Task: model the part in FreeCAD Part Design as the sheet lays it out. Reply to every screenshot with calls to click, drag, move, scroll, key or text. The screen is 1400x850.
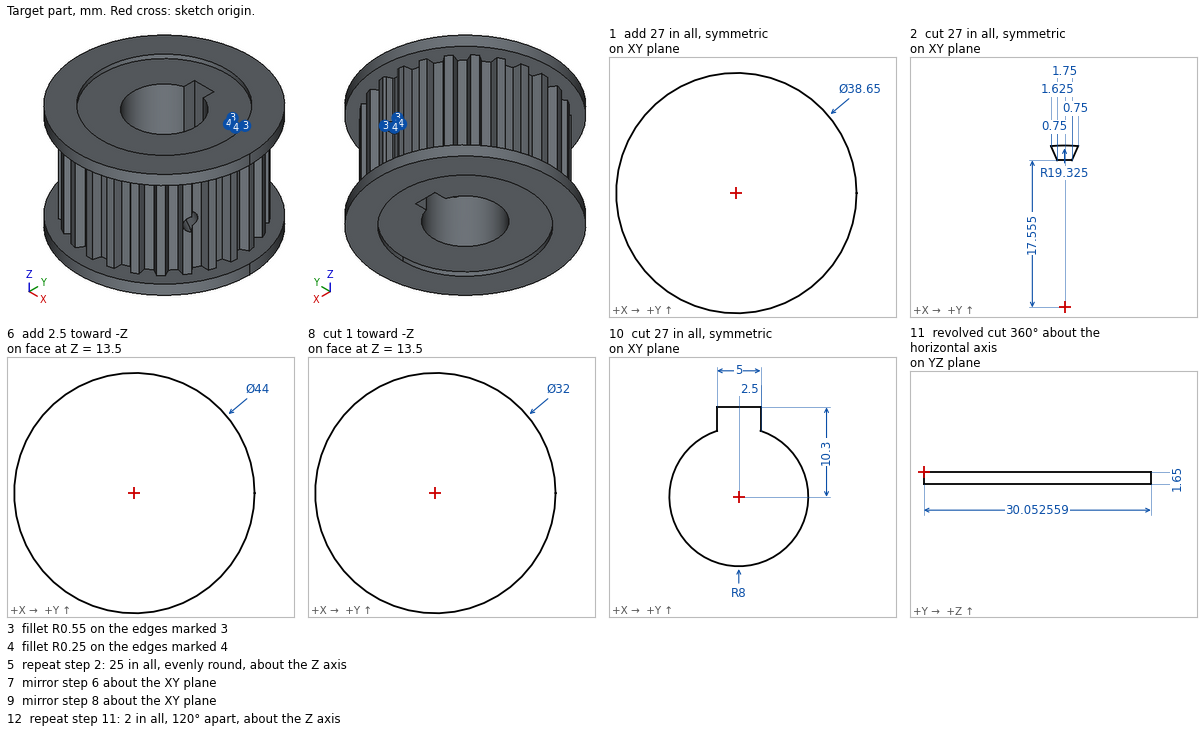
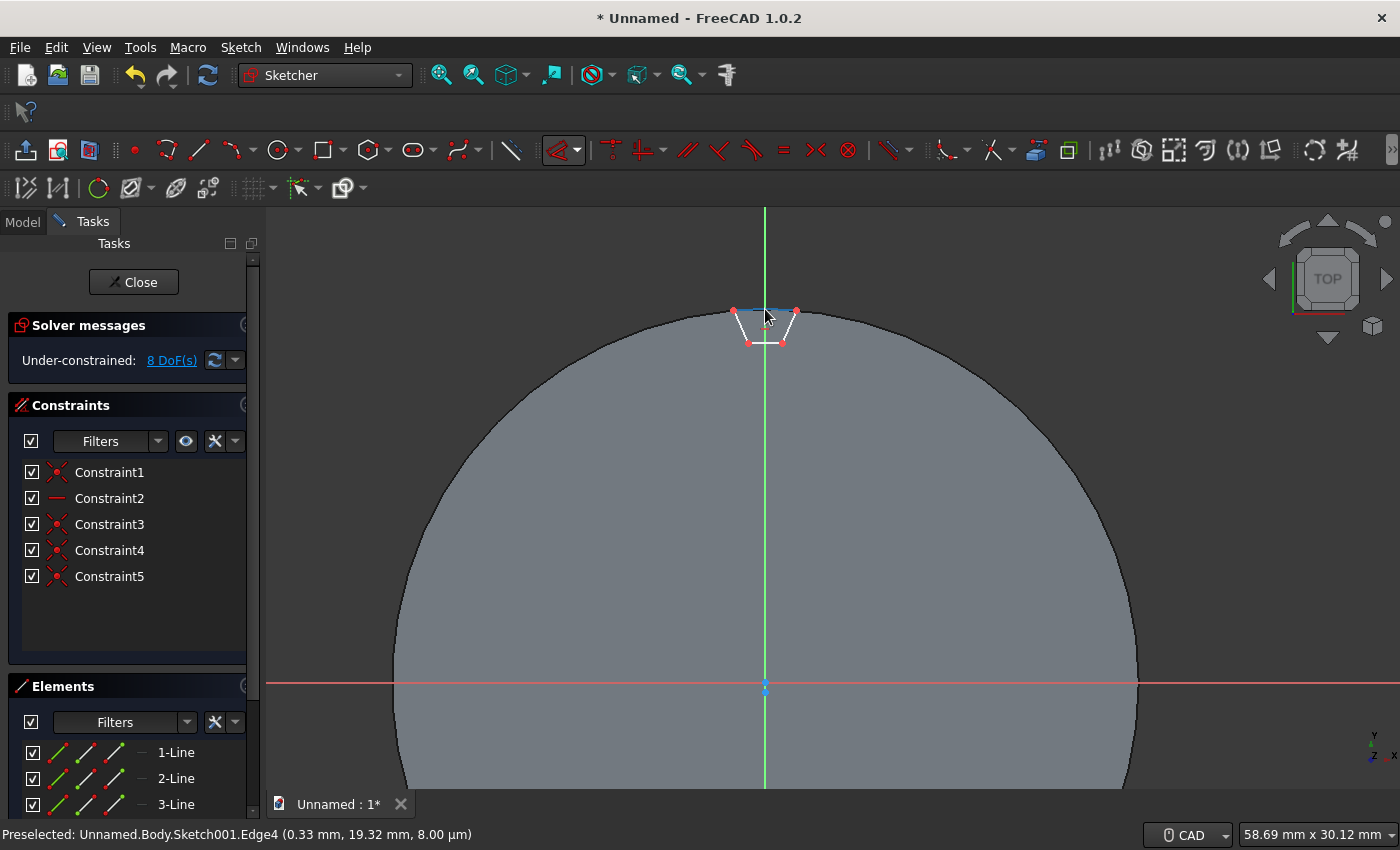
drag(755, 673, 775, 703)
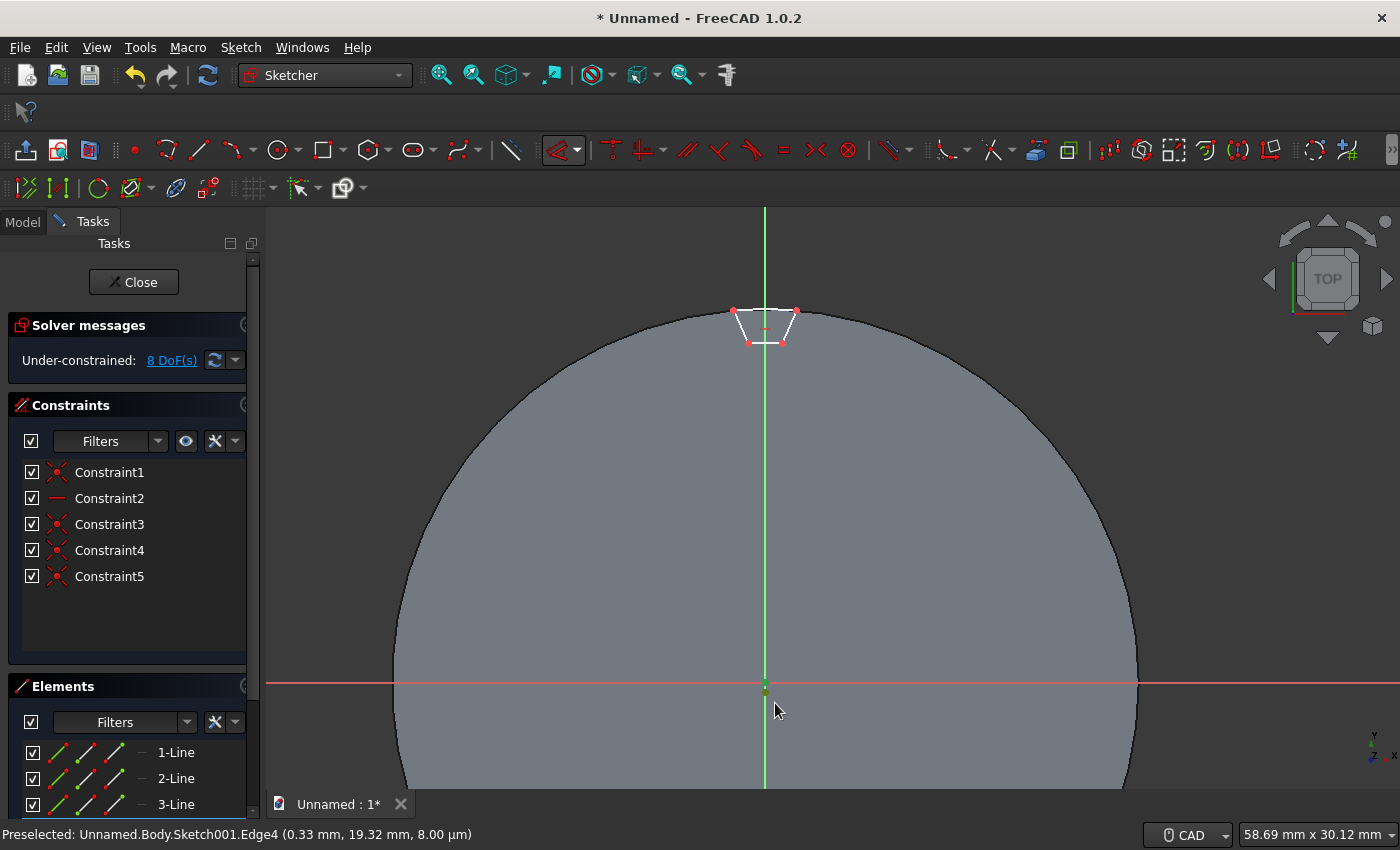
click(612, 150)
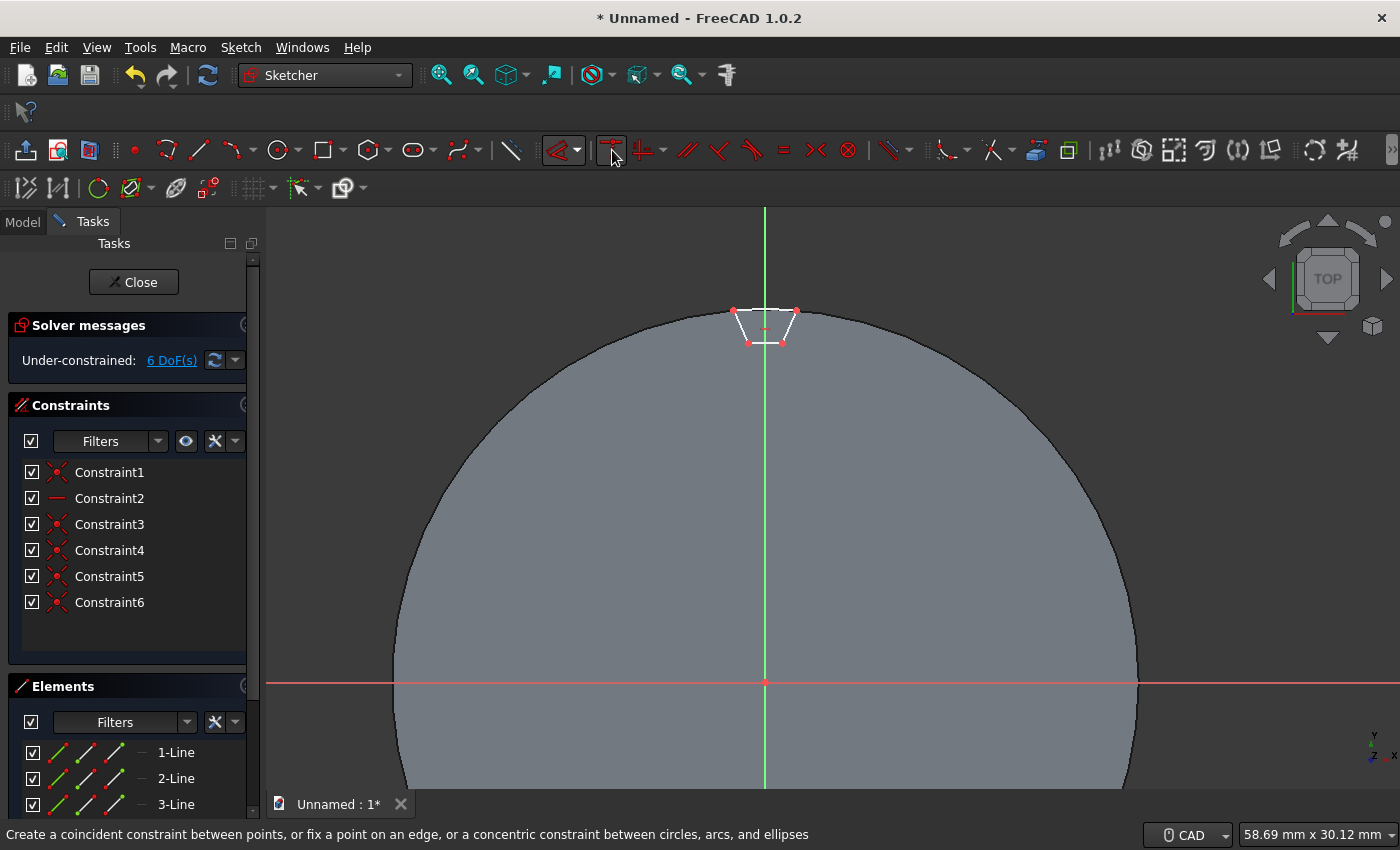
click(558, 150)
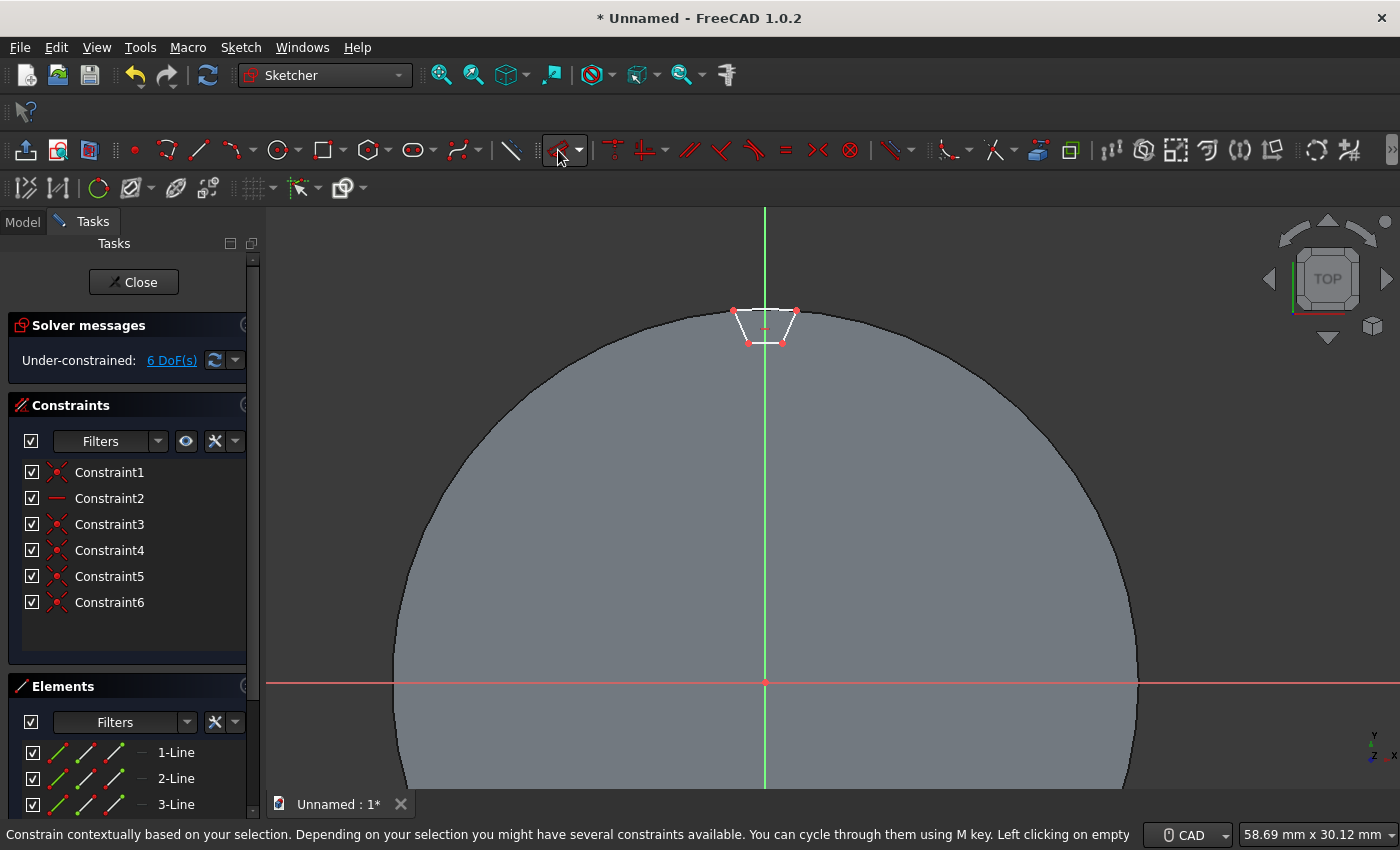
click(778, 309)
click(779, 277)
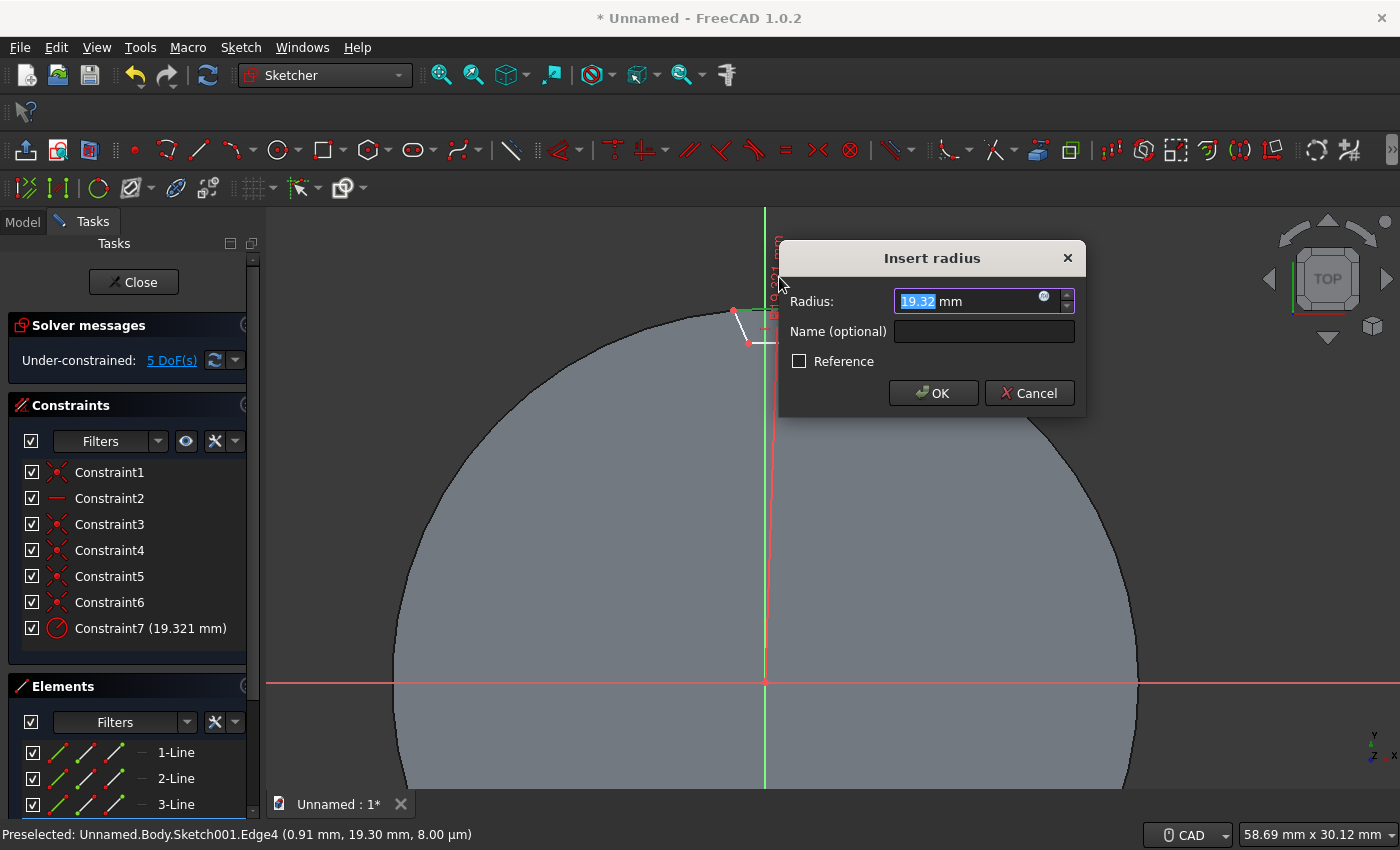
text(19.325)
key(Return)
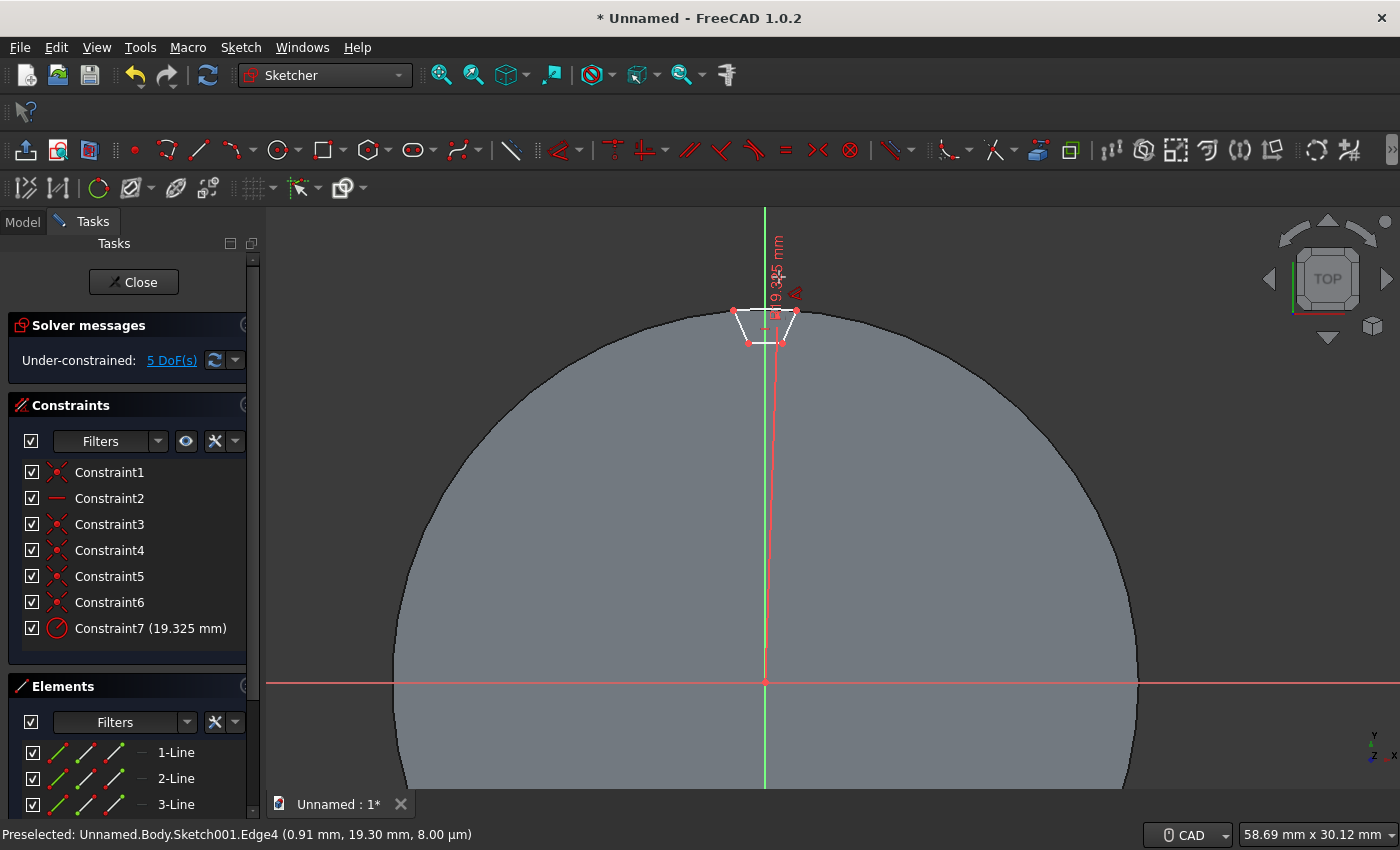
click(762, 343)
click(758, 377)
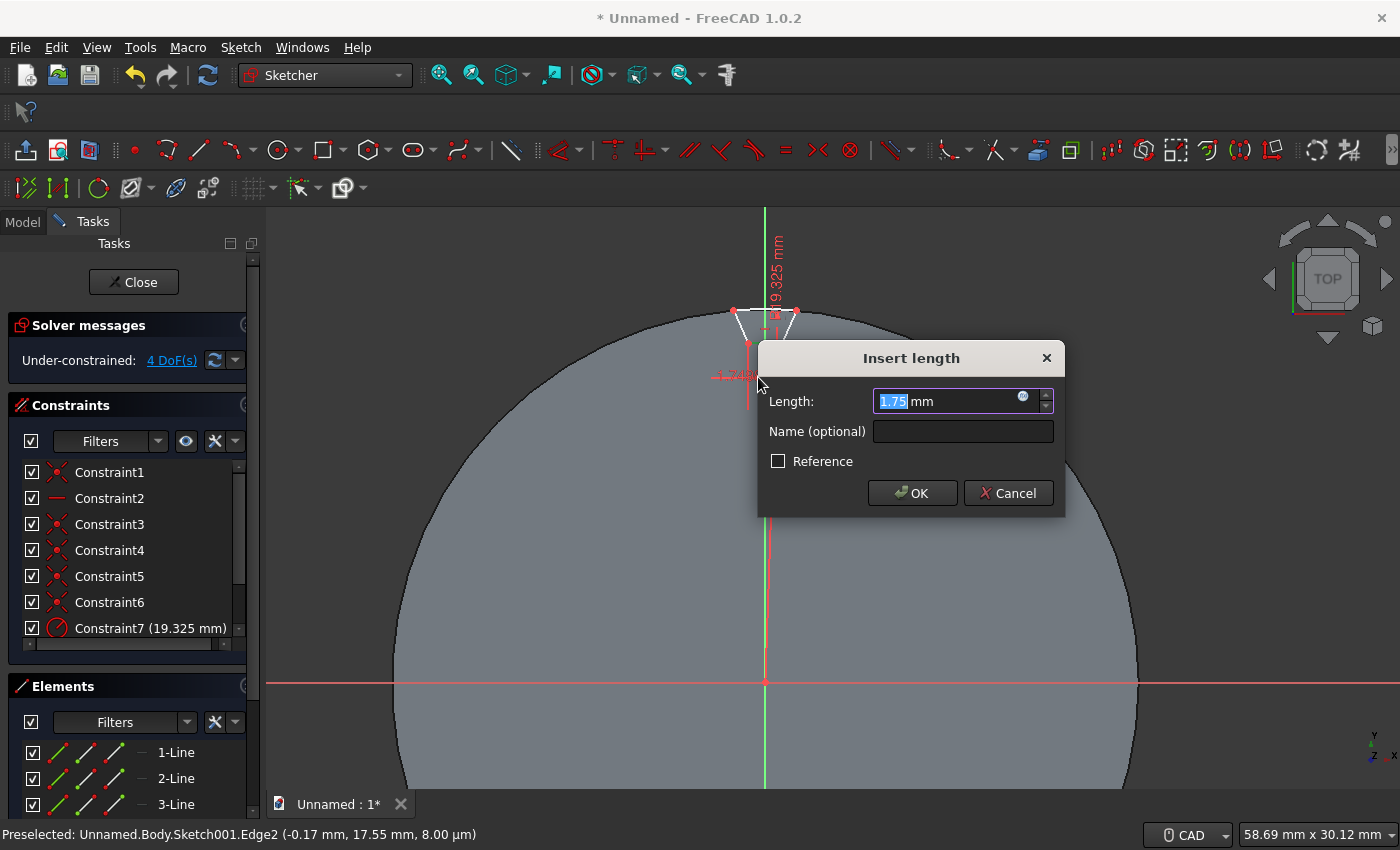
text(1.75)
key(Return)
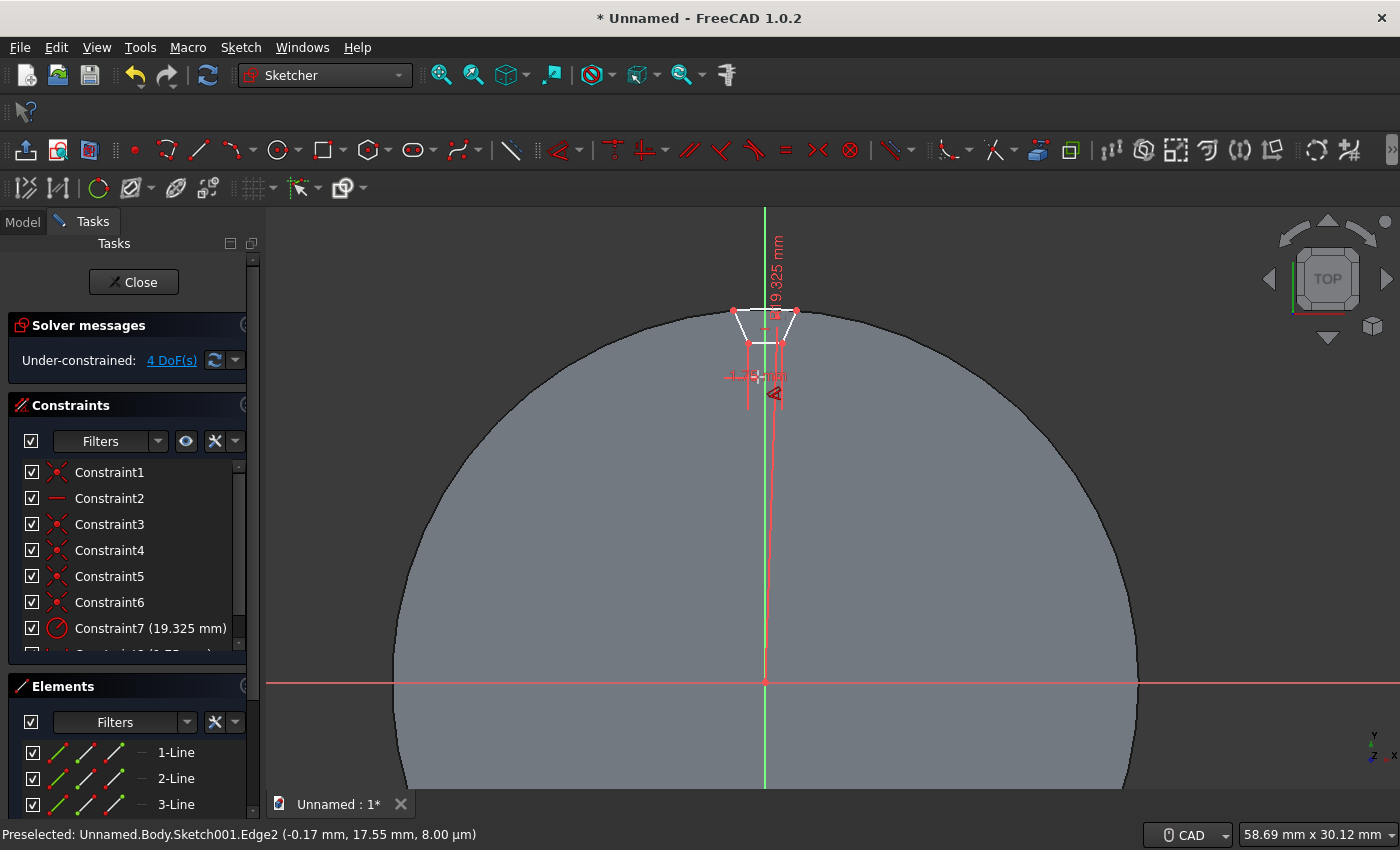
scroll(738, 320, up, 6)